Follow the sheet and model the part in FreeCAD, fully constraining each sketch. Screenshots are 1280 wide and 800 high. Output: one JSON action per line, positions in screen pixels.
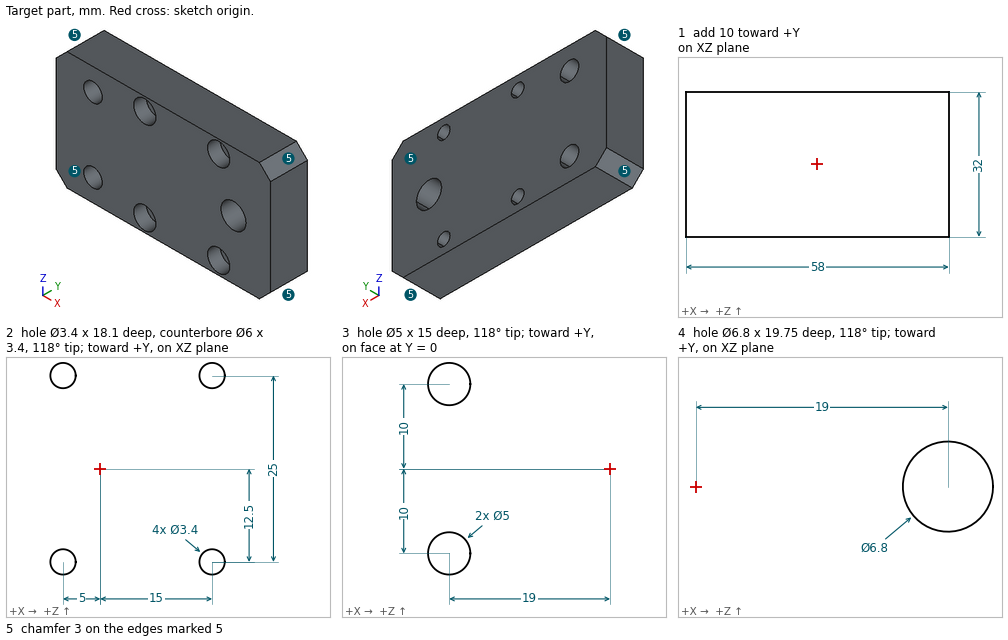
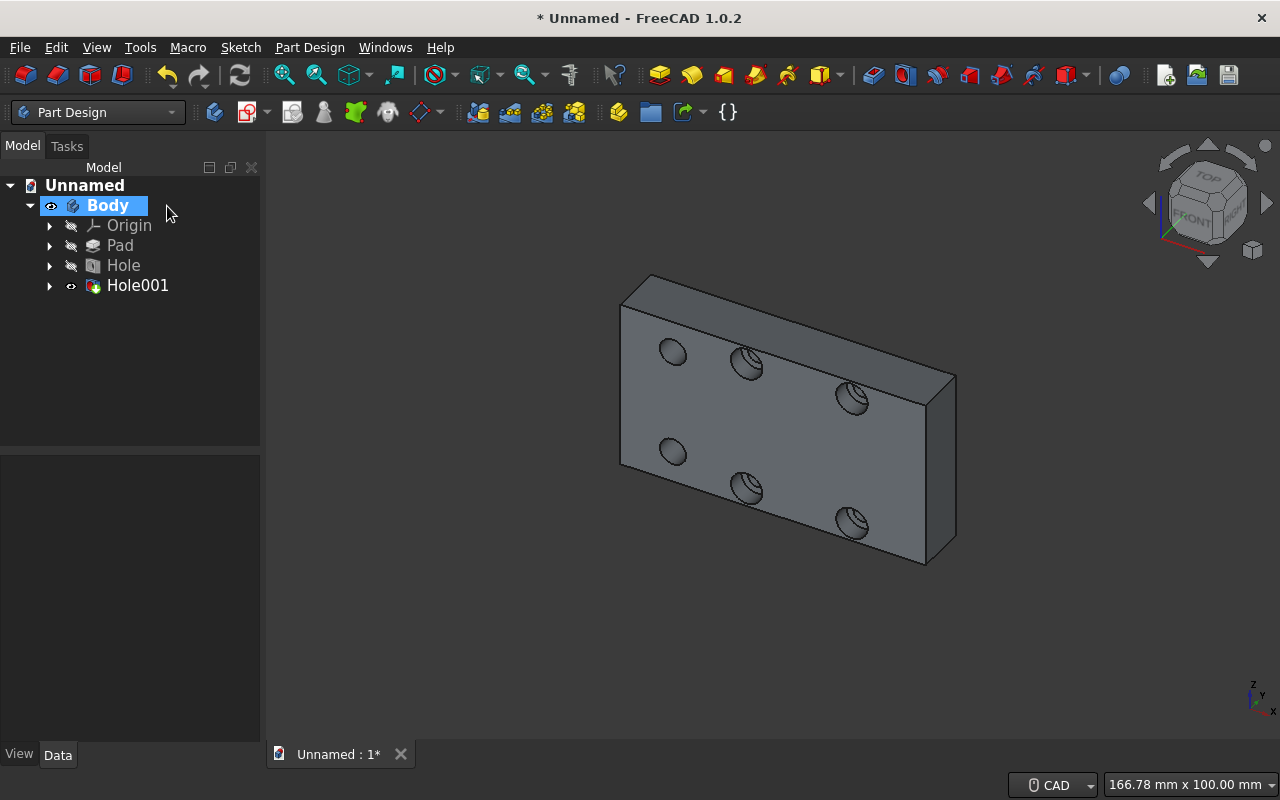
{"action": "left_click", "coordinate": [248, 112]}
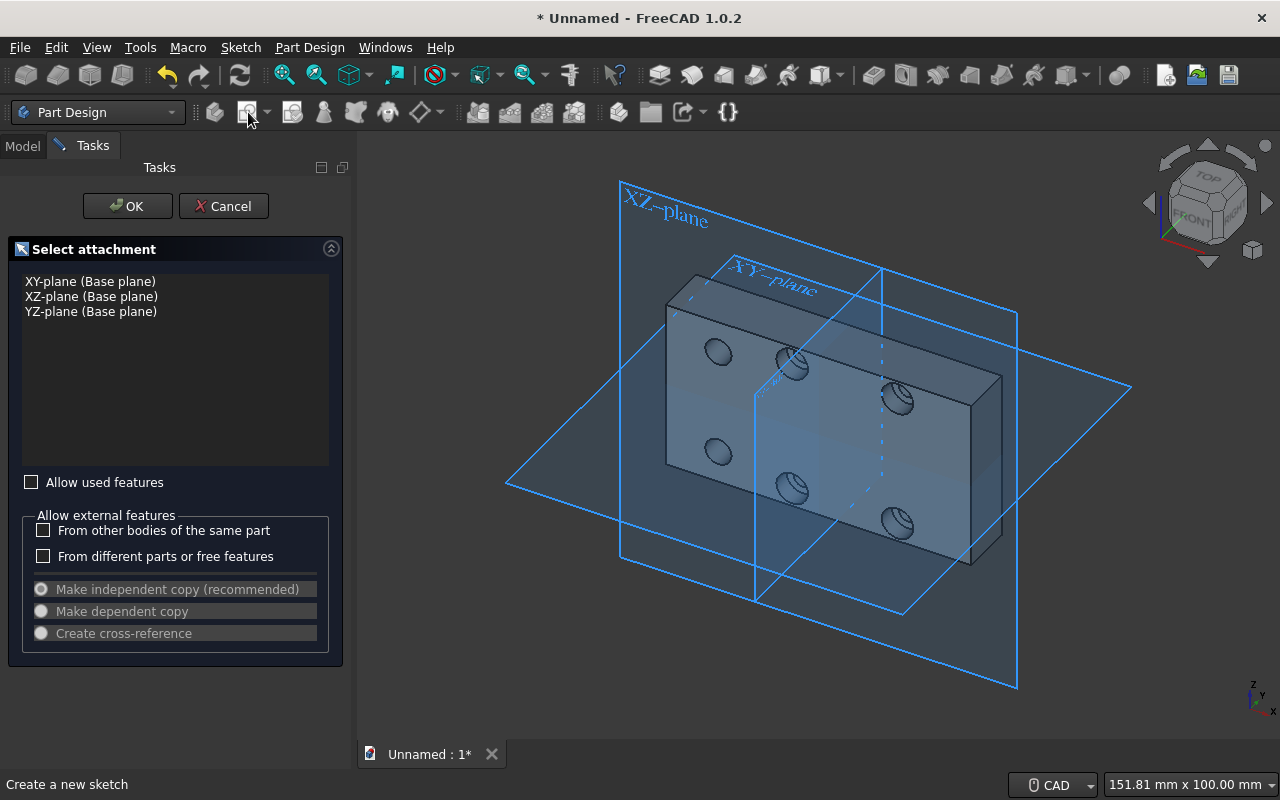
{"action": "left_click", "coordinate": [82, 296]}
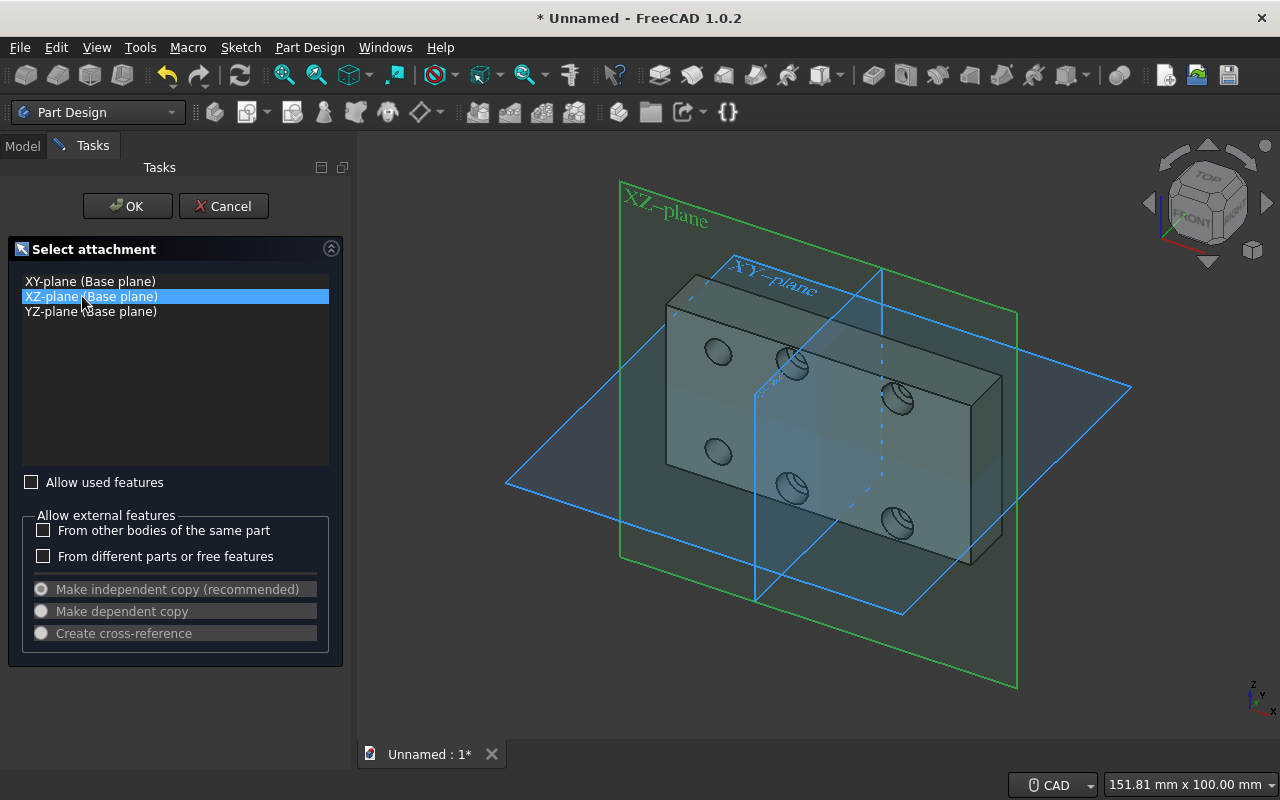
{"action": "left_click", "coordinate": [128, 206]}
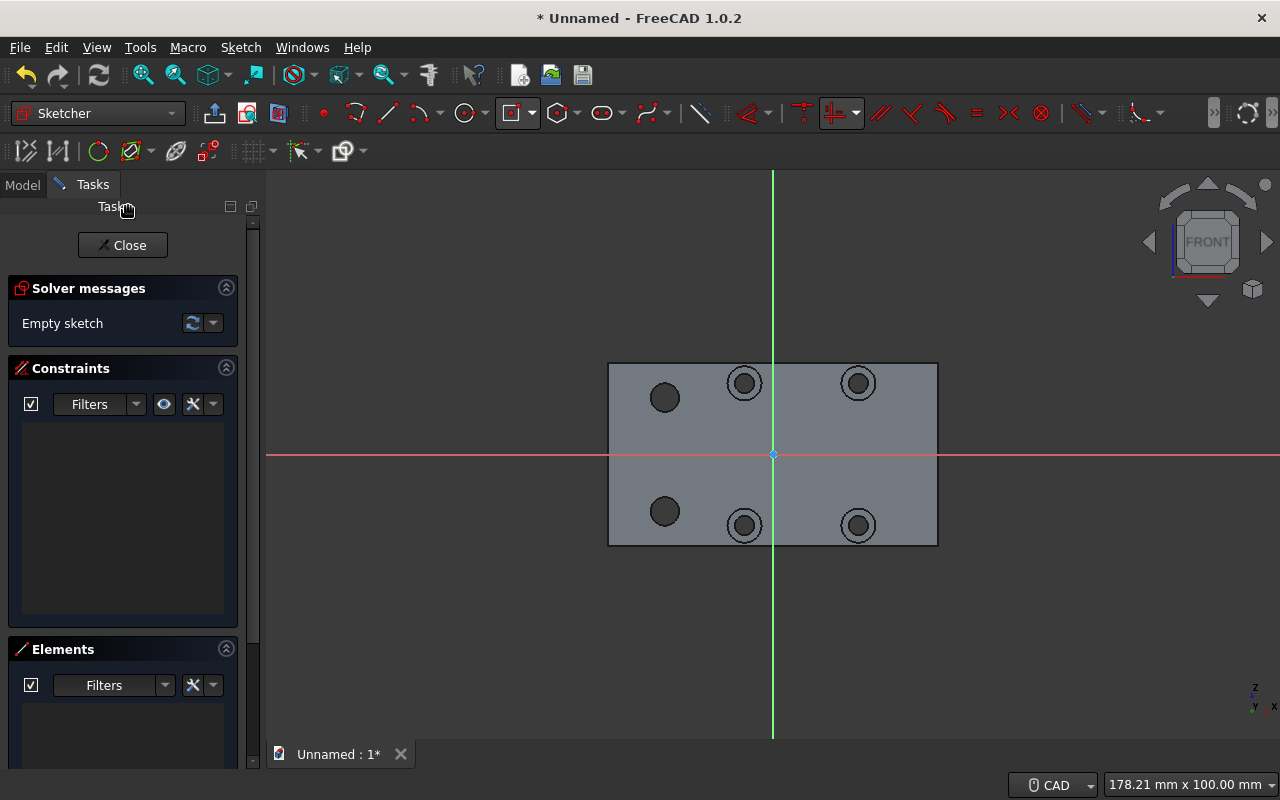
{"action": "scroll", "coordinate": [903, 454], "scroll_direction": "up", "scroll_amount": 11}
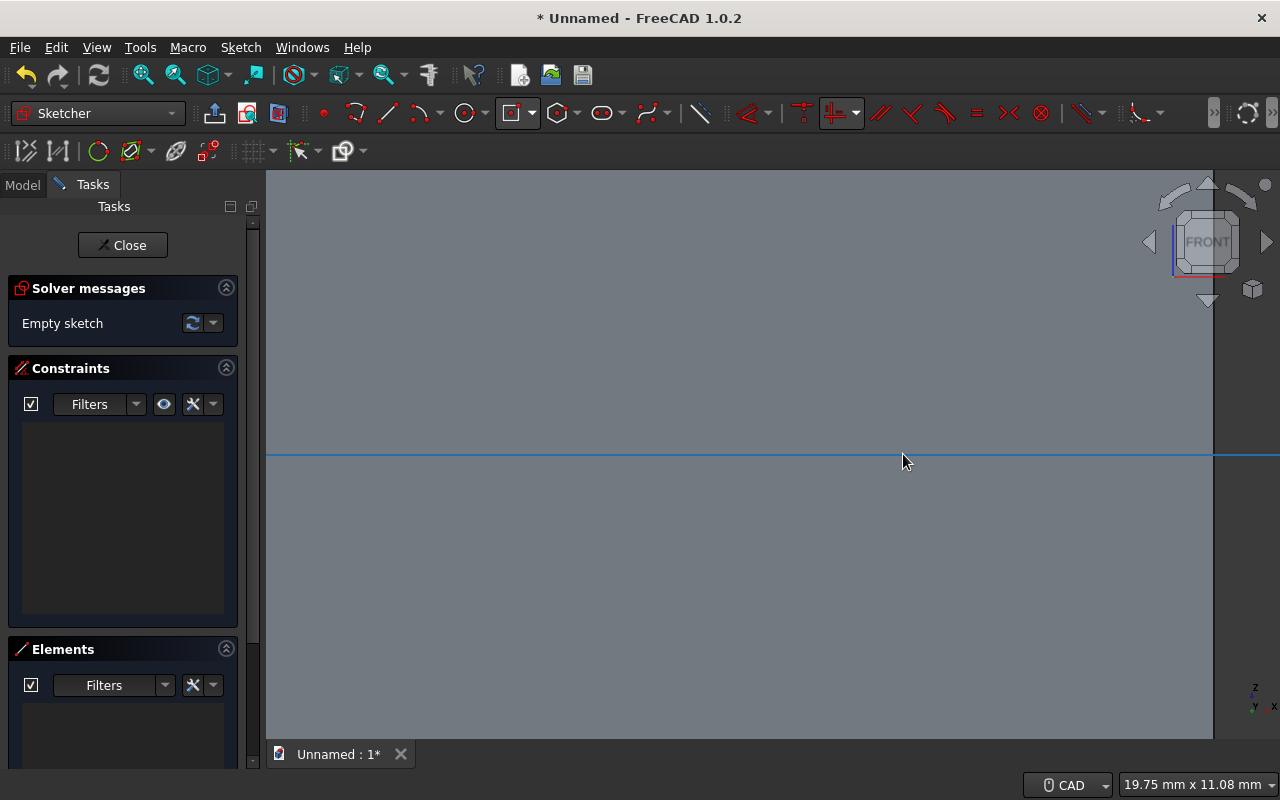
{"action": "left_click", "coordinate": [466, 114]}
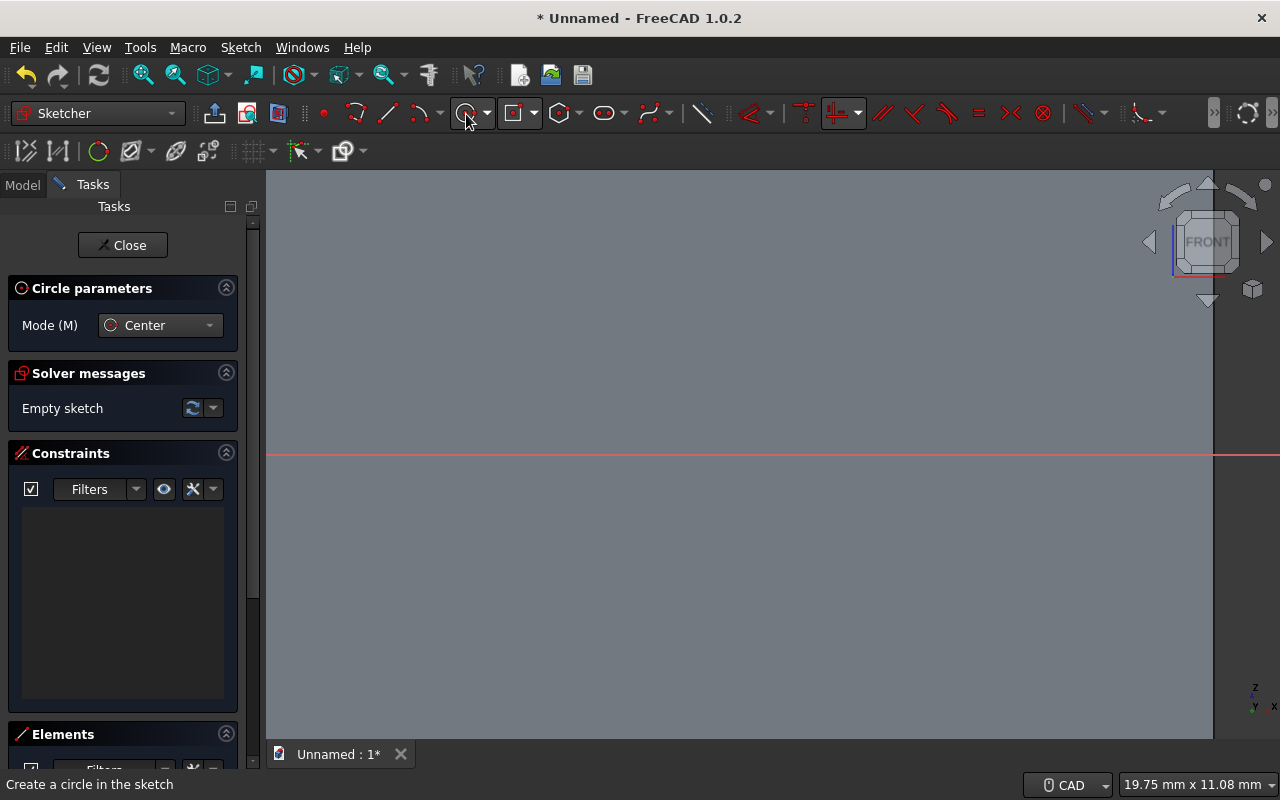
{"action": "left_click", "coordinate": [700, 454]}
{"action": "left_click", "coordinate": [824, 331]}
{"action": "key", "text": "Escape"}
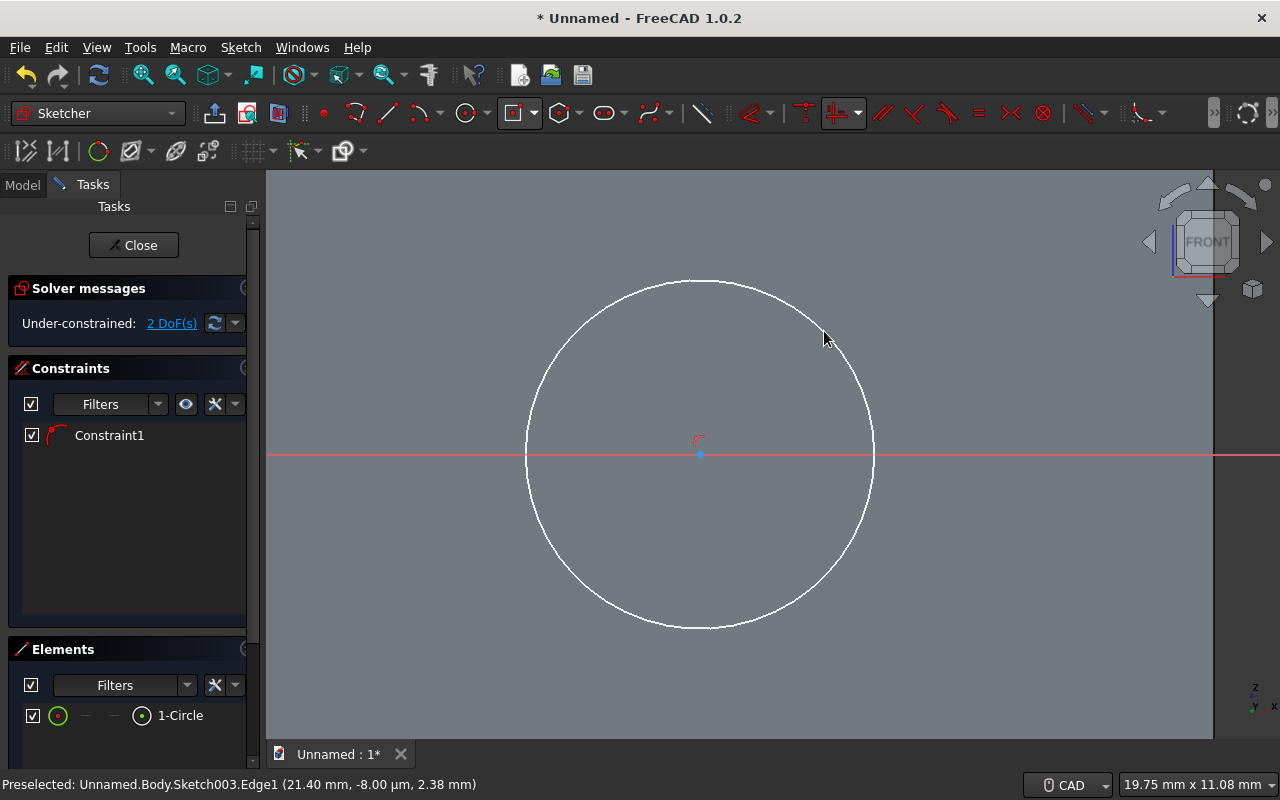
{"action": "left_click", "coordinate": [750, 114]}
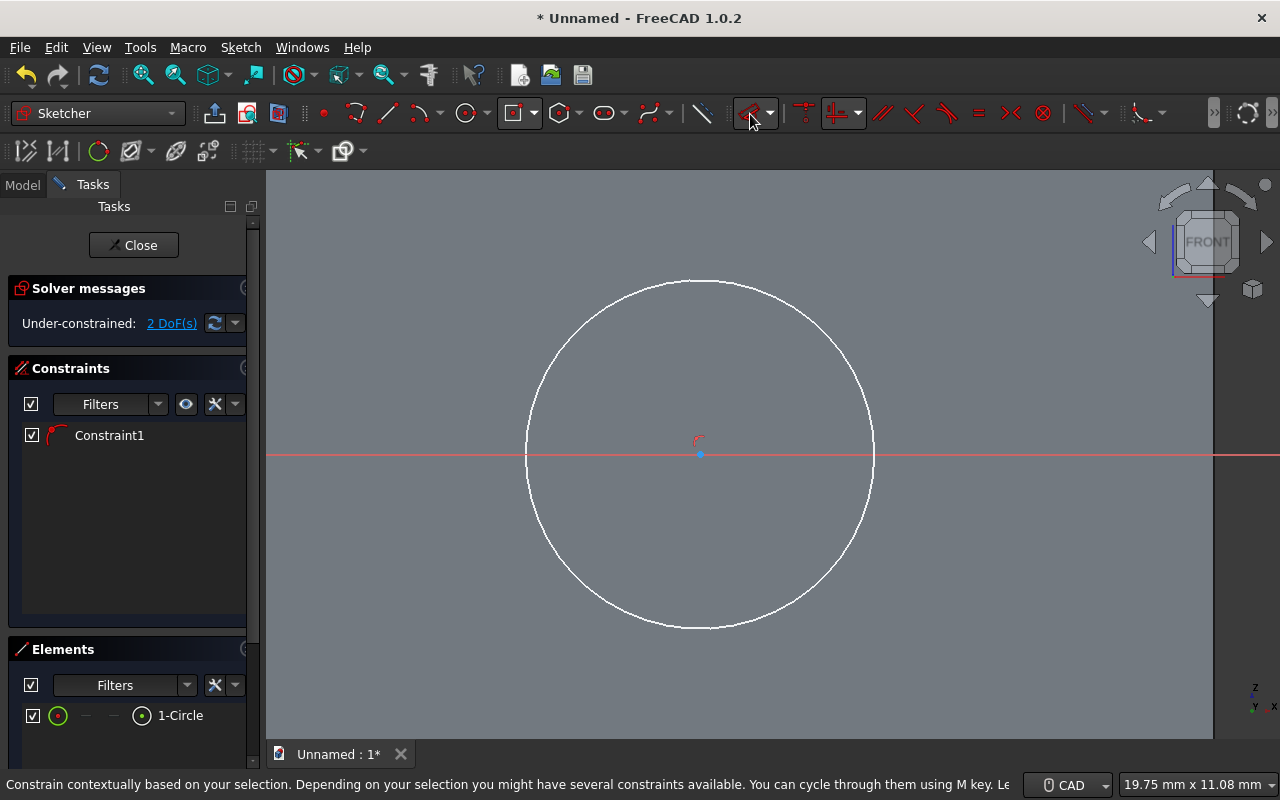
{"action": "left_click", "coordinate": [823, 331]}
{"action": "left_click", "coordinate": [846, 308]}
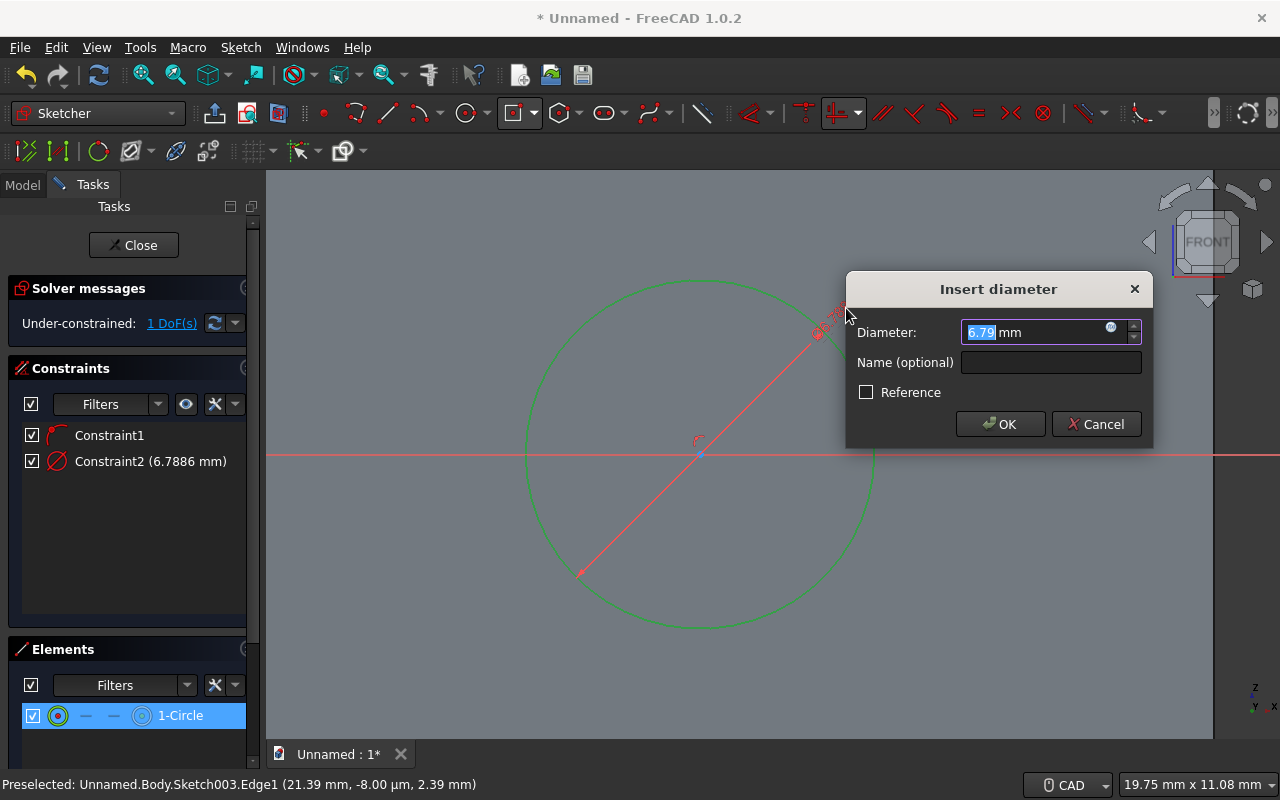
{"action": "type", "text": "6.8"}
{"action": "key", "text": "Return"}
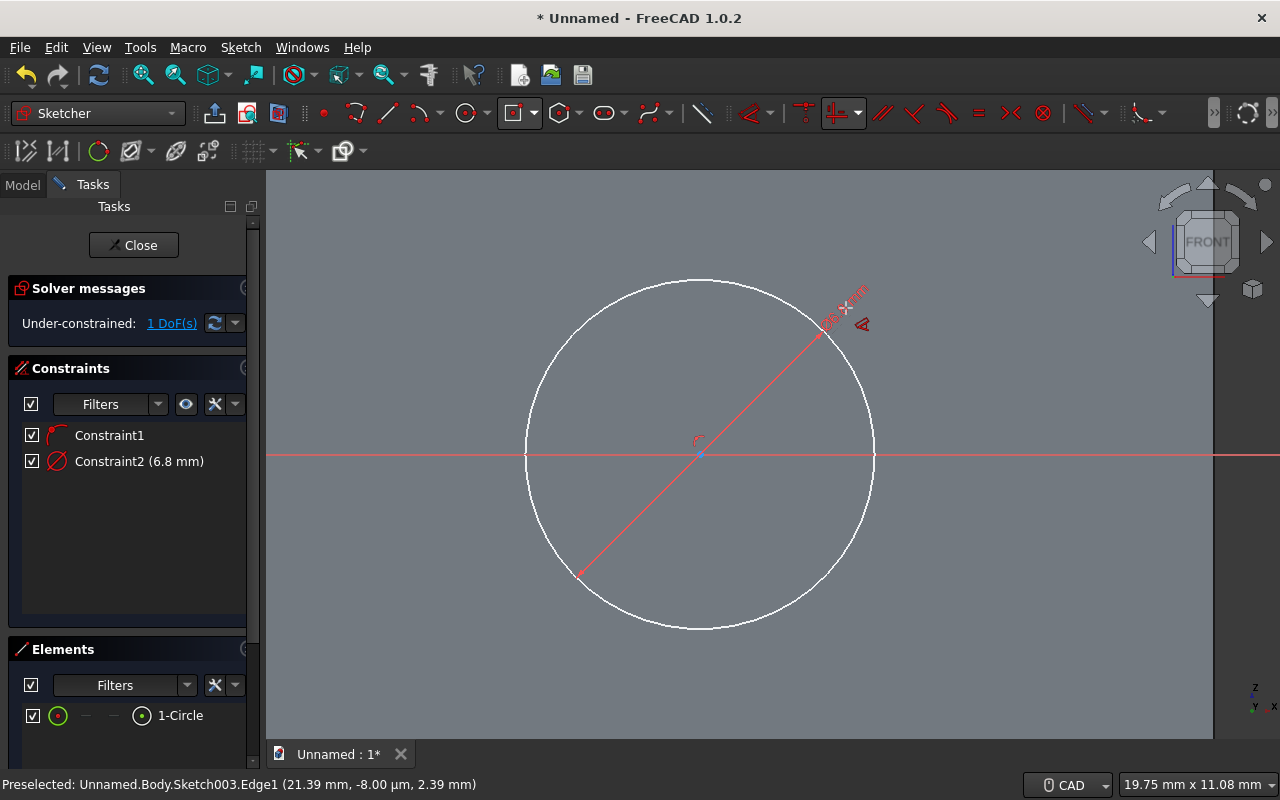
{"action": "left_click", "coordinate": [700, 454]}
{"action": "left_click", "coordinate": [497, 488]}